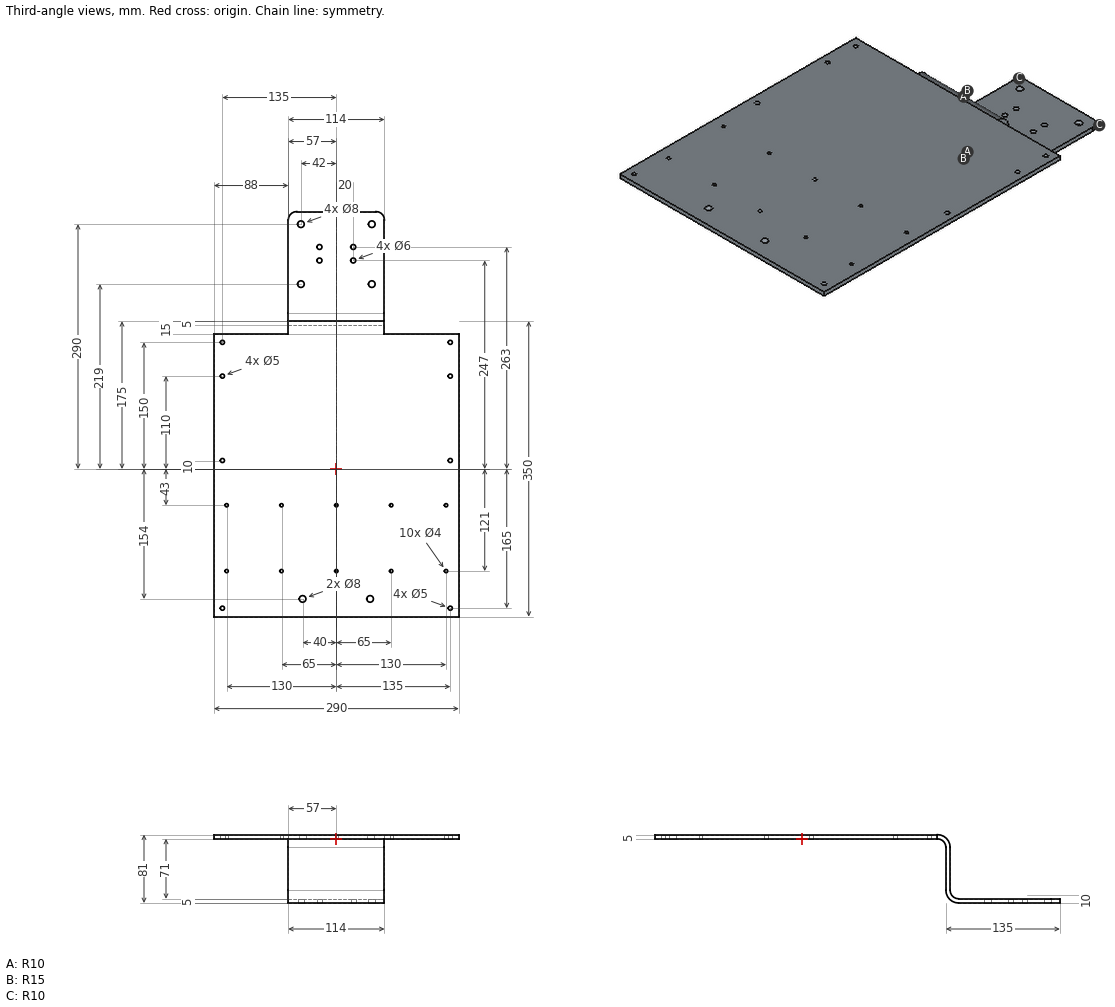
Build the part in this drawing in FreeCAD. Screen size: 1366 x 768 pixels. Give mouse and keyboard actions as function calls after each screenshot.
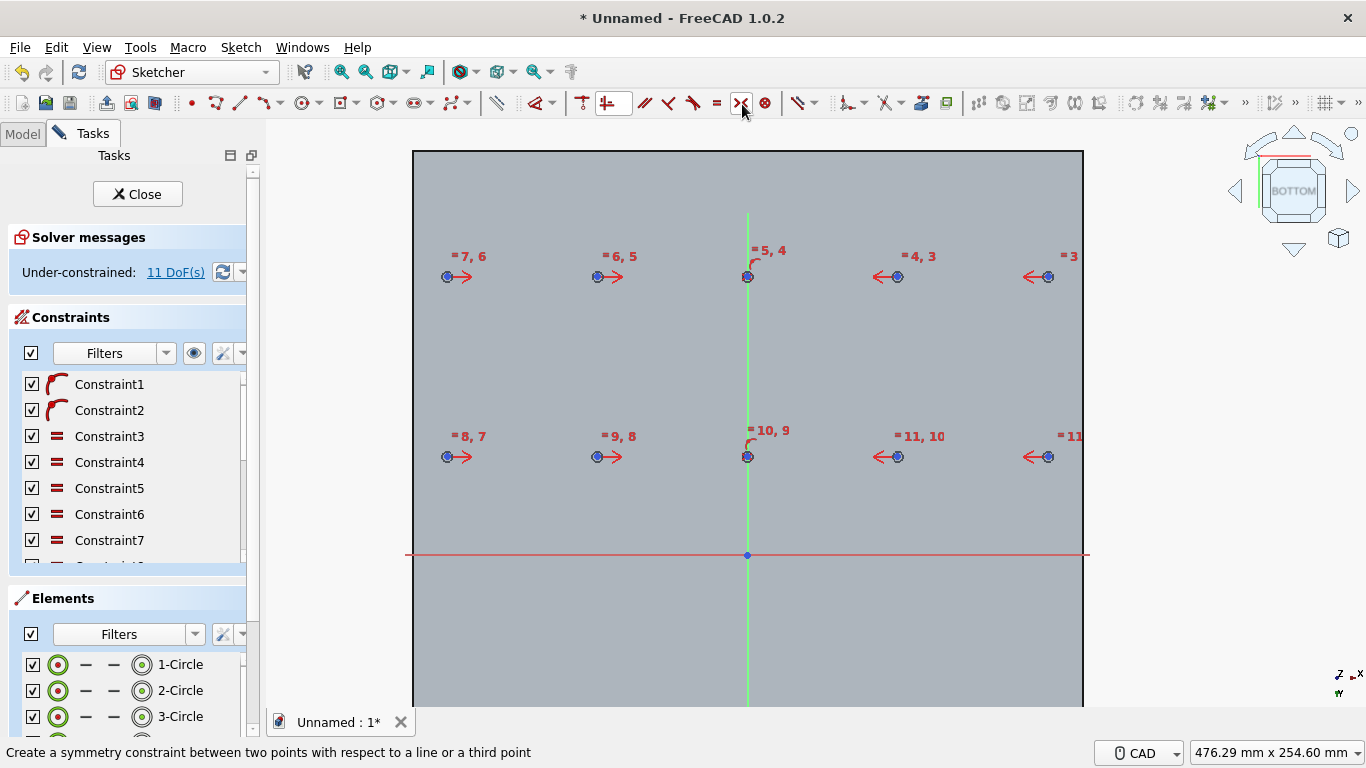
click(536, 104)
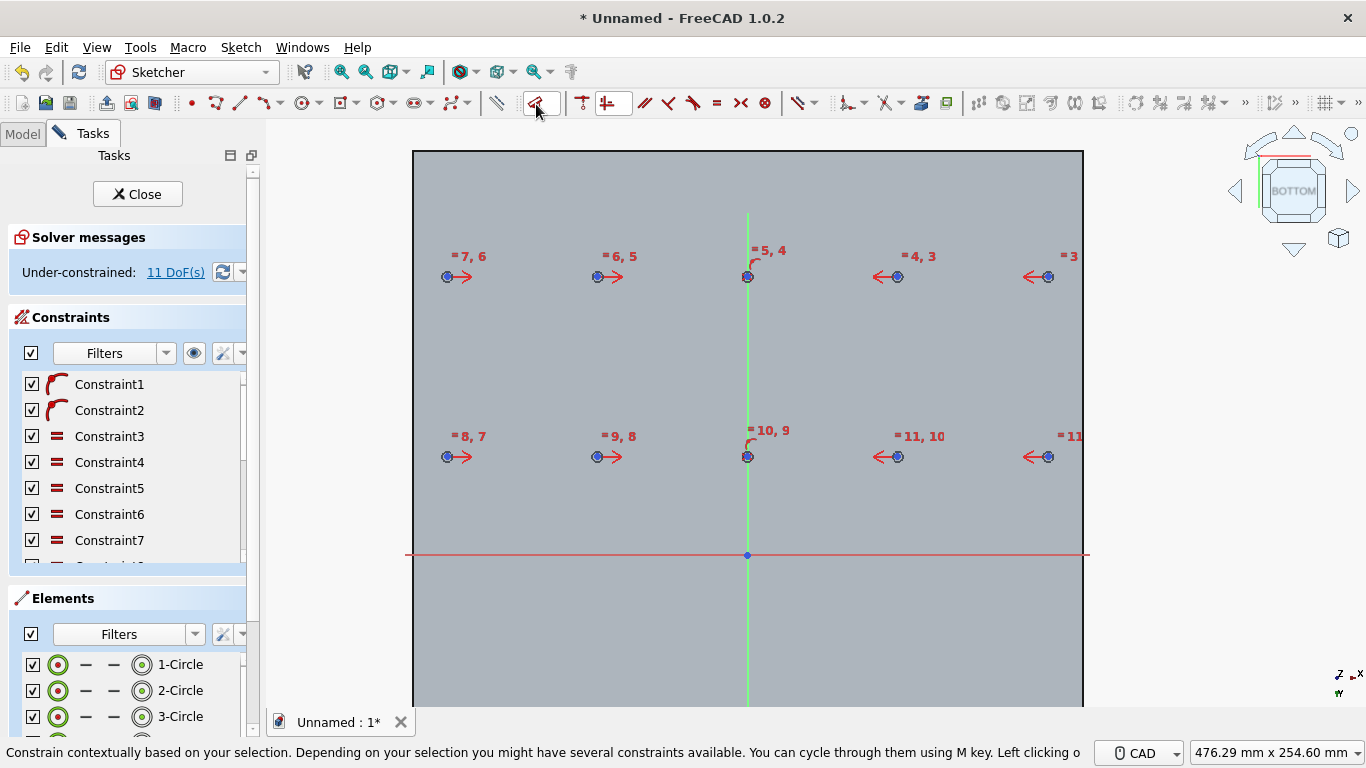
scroll(1045, 273, up, 8)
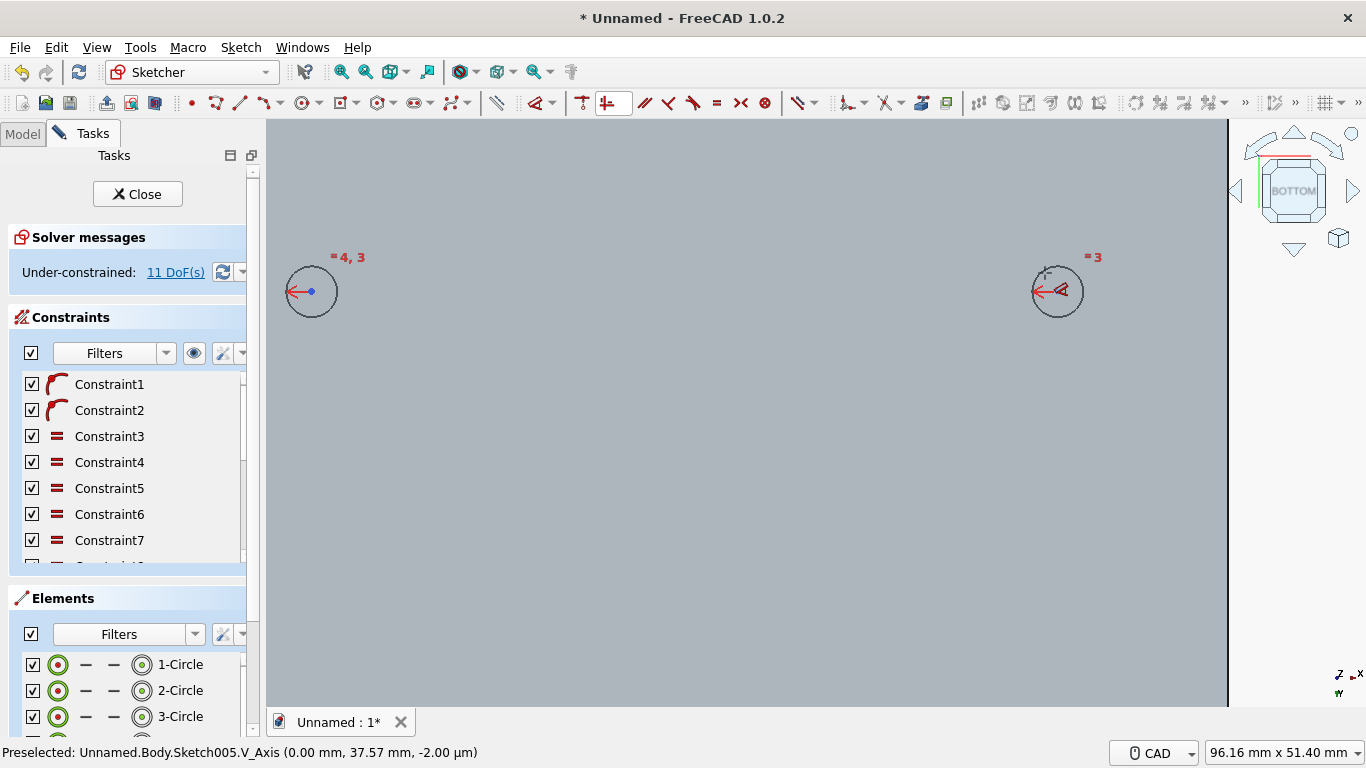
click(1040, 274)
click(1017, 251)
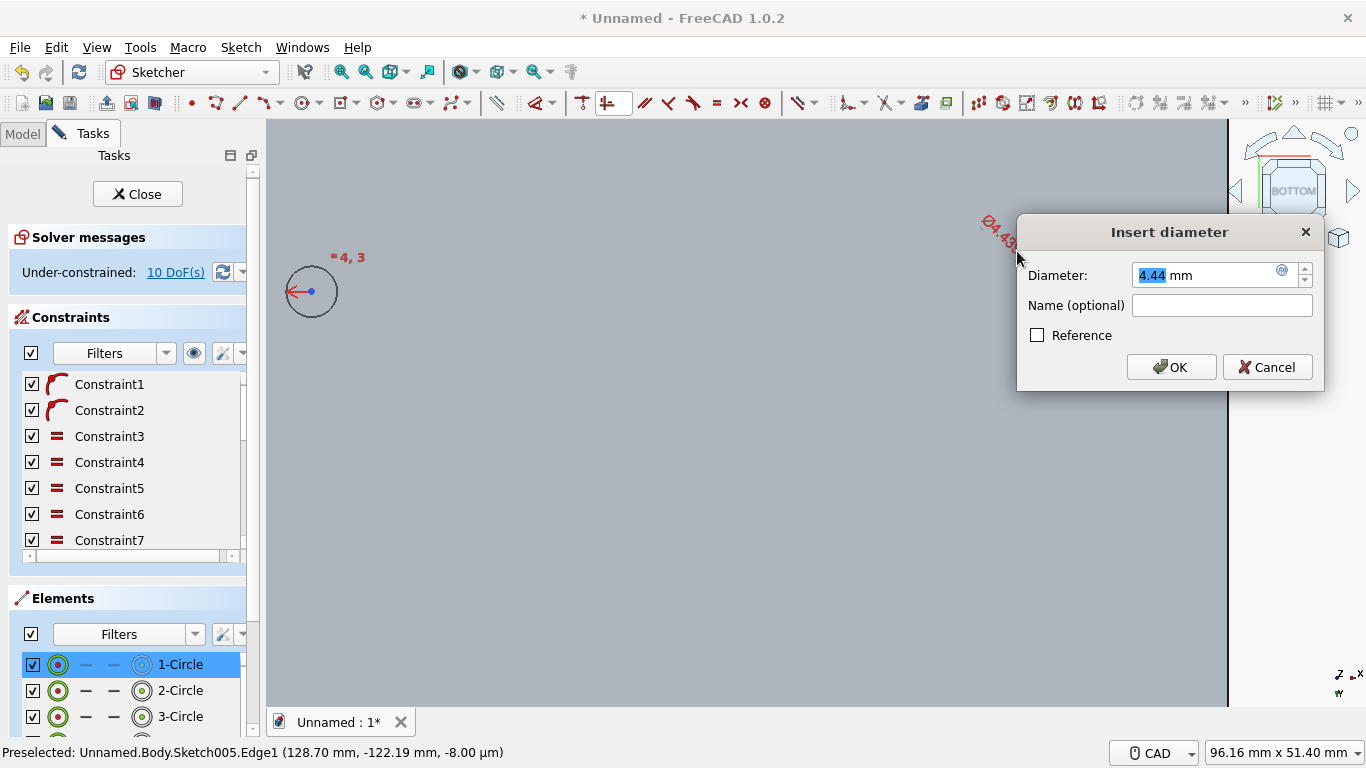
text(4)
key(Return)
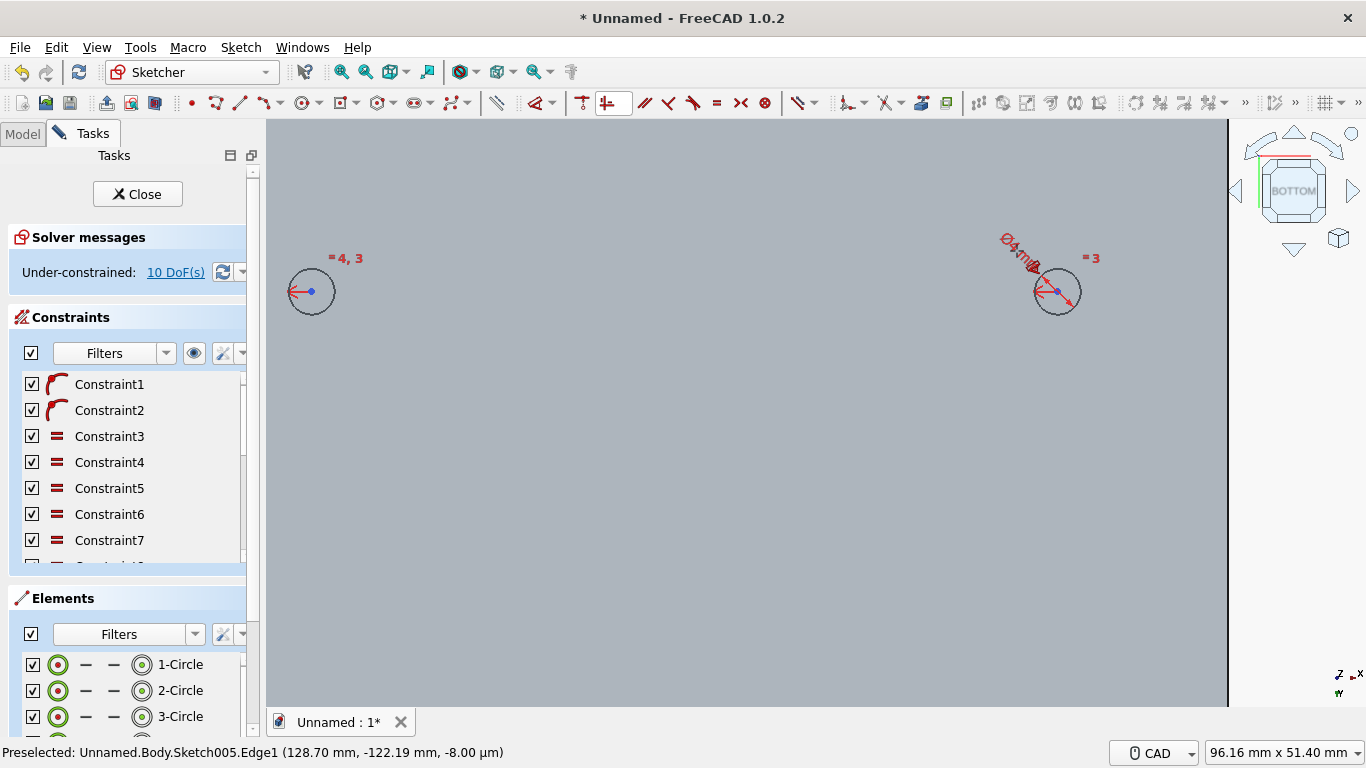
scroll(1046, 273, down, 8)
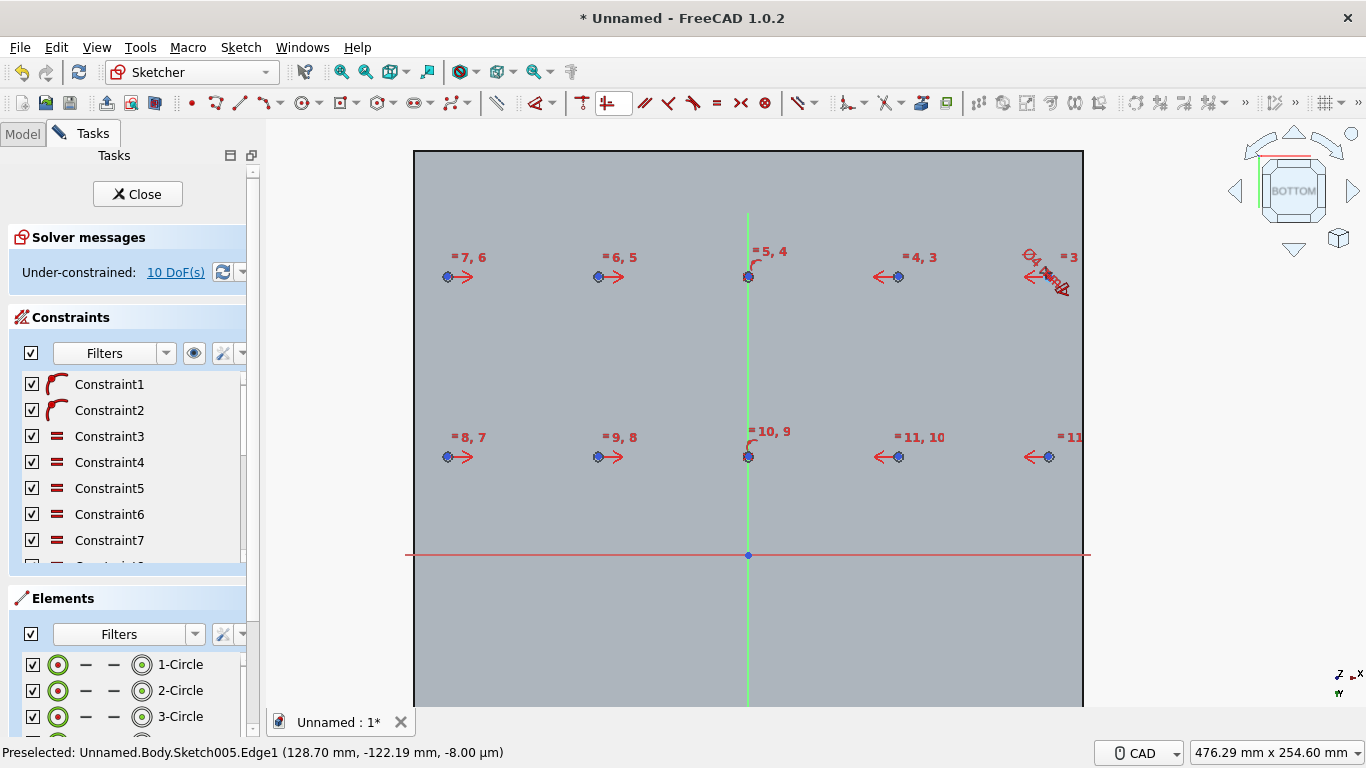
click(898, 277)
click(823, 589)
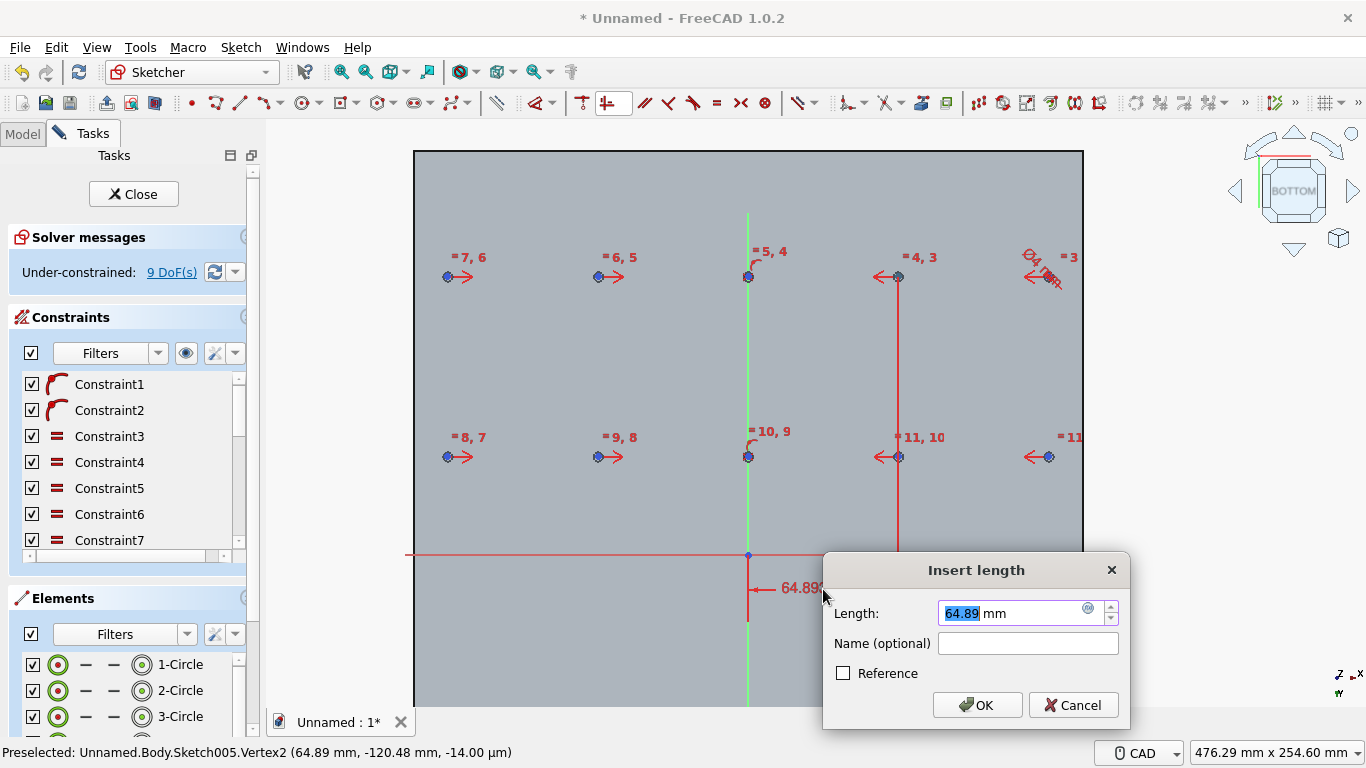
text(65)
key(Return)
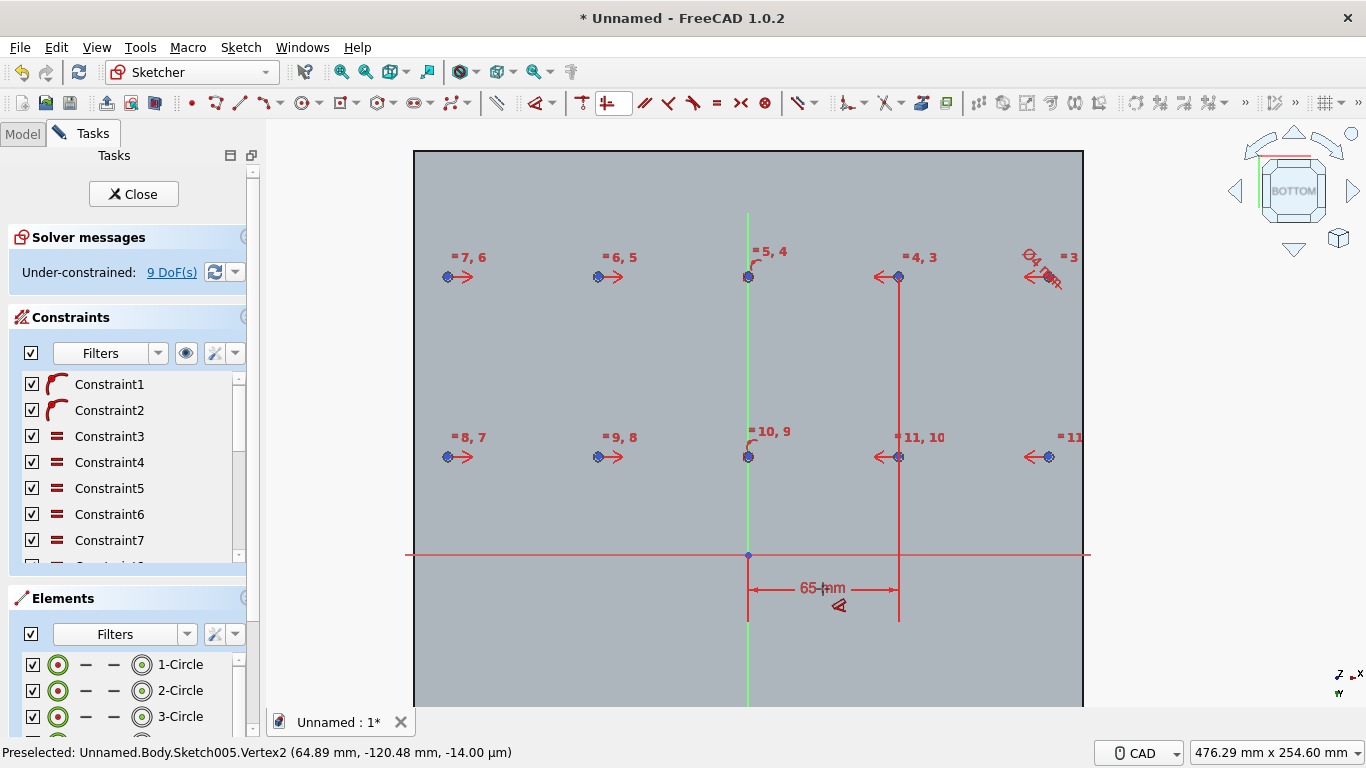
click(448, 457)
click(414, 506)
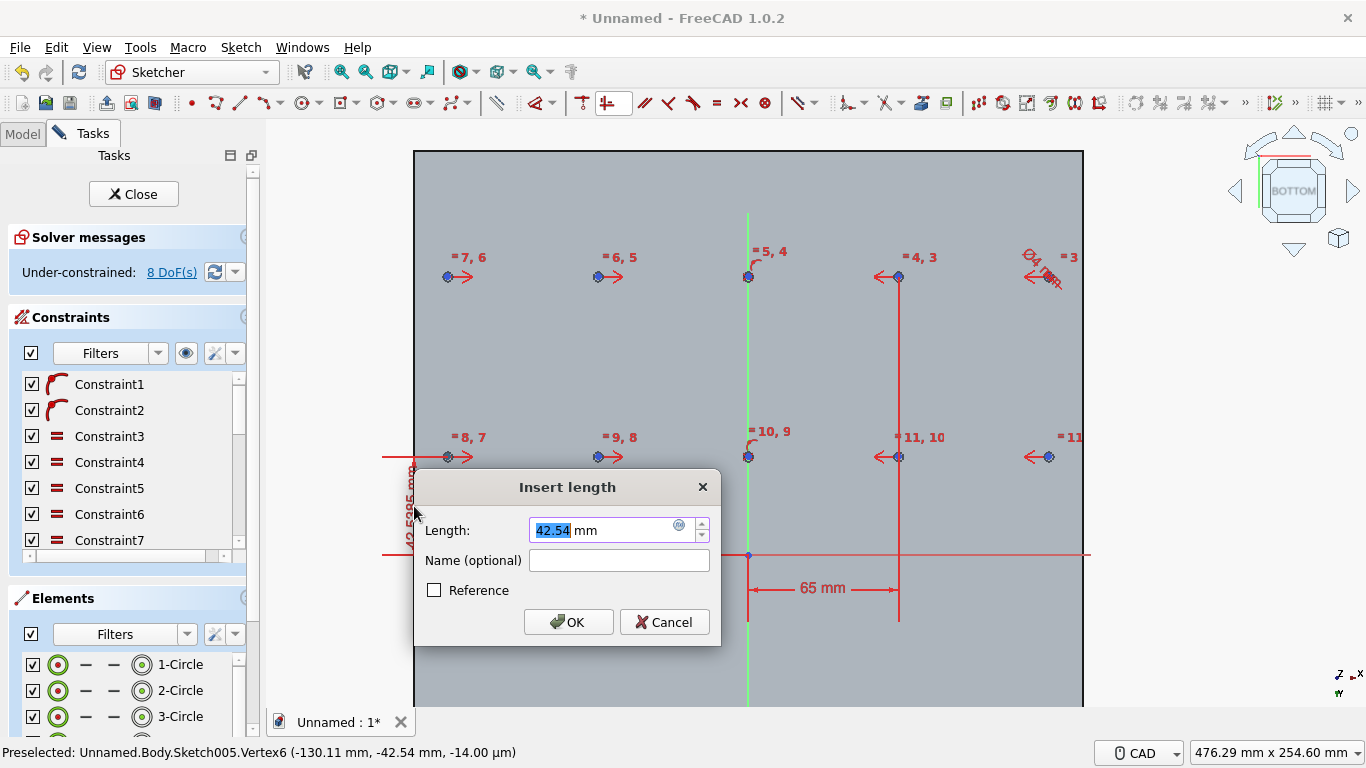
text(43)
key(Return)